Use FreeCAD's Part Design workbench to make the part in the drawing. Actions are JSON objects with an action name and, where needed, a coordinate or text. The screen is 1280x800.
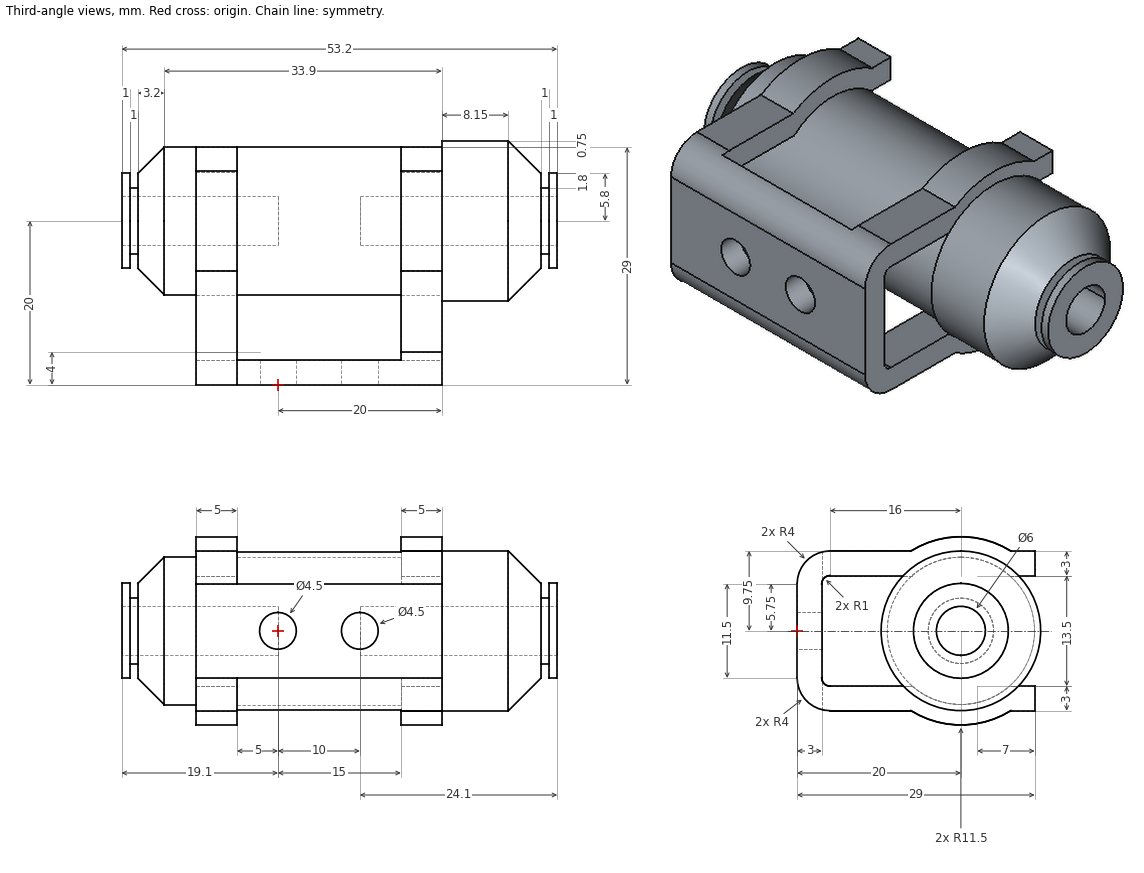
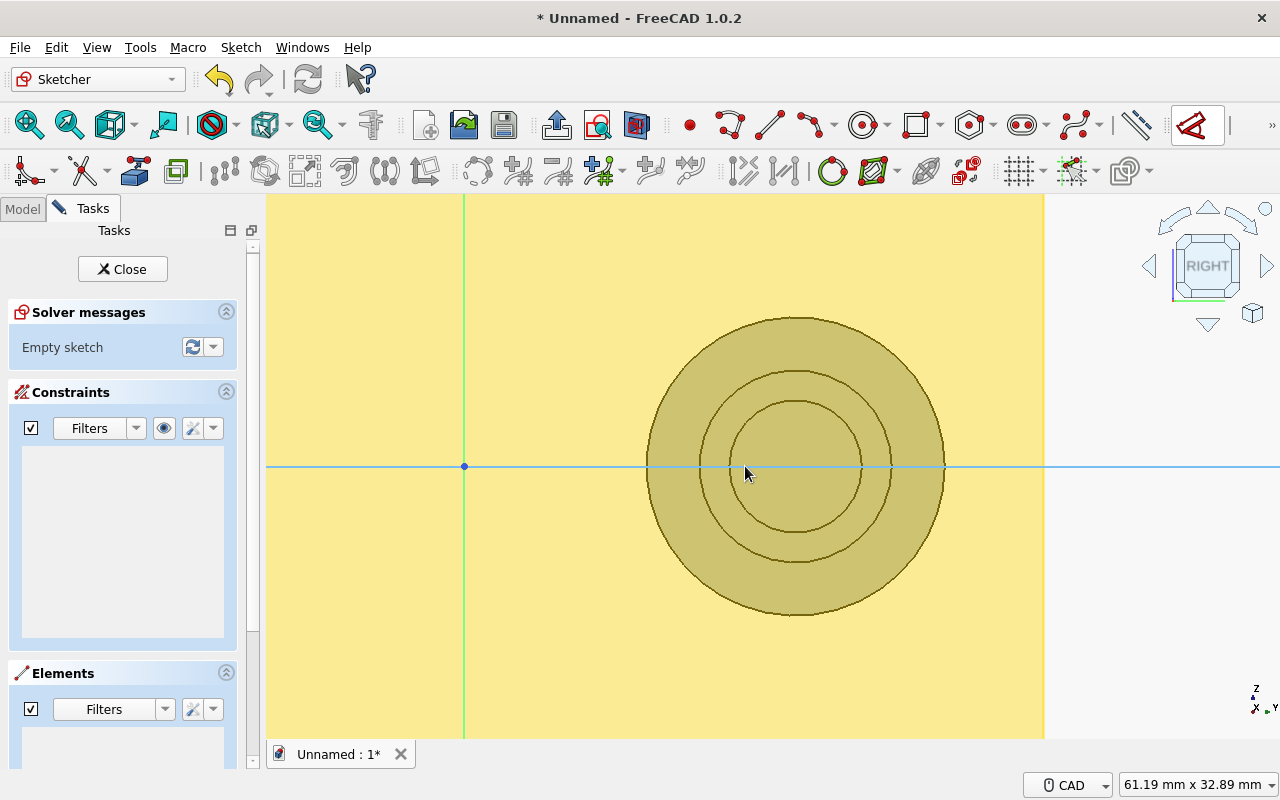
{"action": "left_click", "coordinate": [770, 126]}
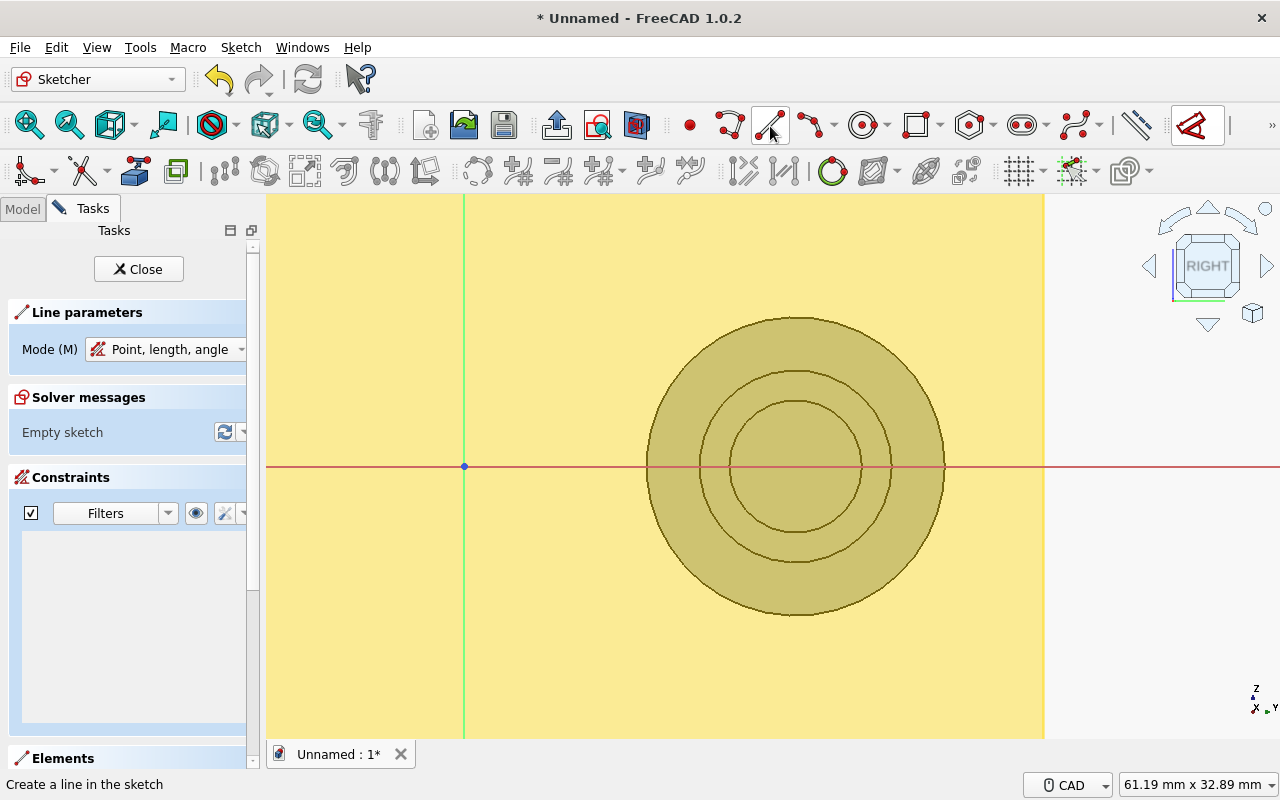
{"action": "left_click", "coordinate": [695, 305]}
{"action": "left_click", "coordinate": [530, 305]}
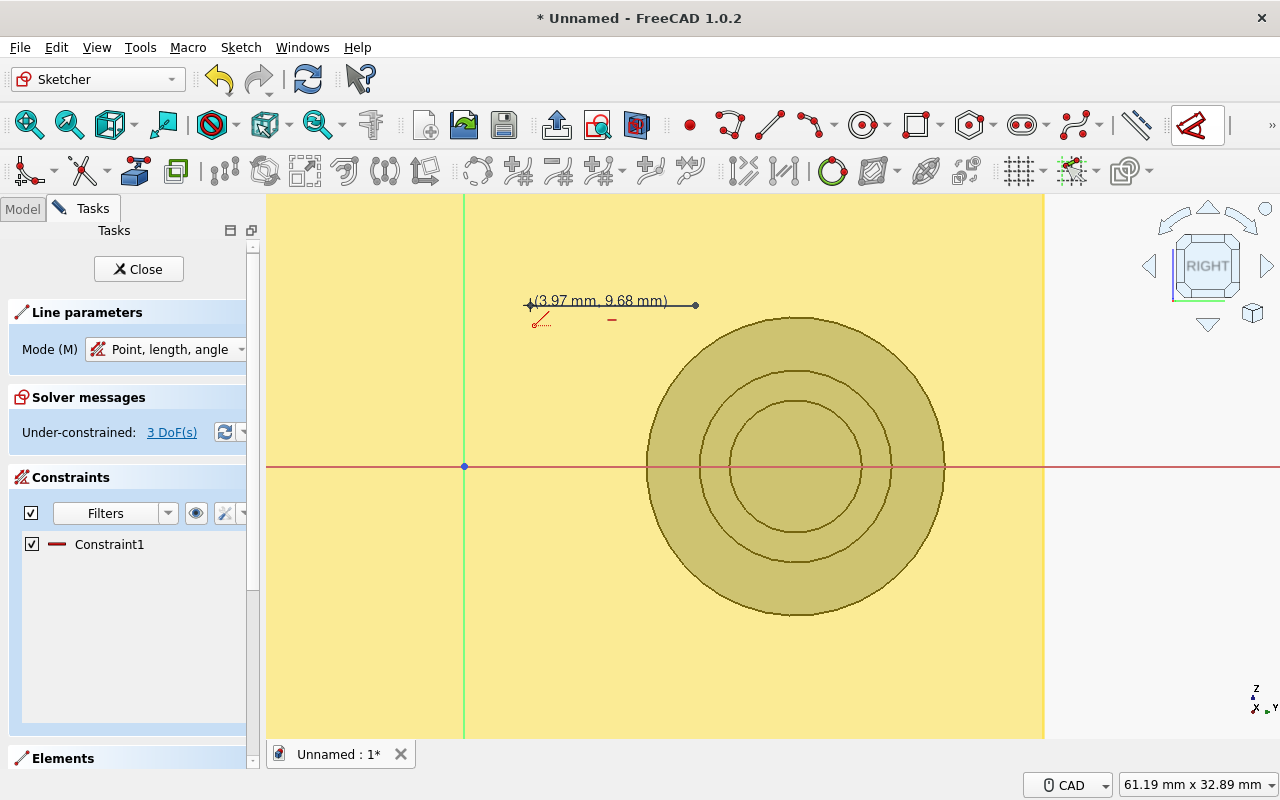
{"action": "left_click", "coordinate": [464, 371]}
{"action": "left_click", "coordinate": [473, 562]}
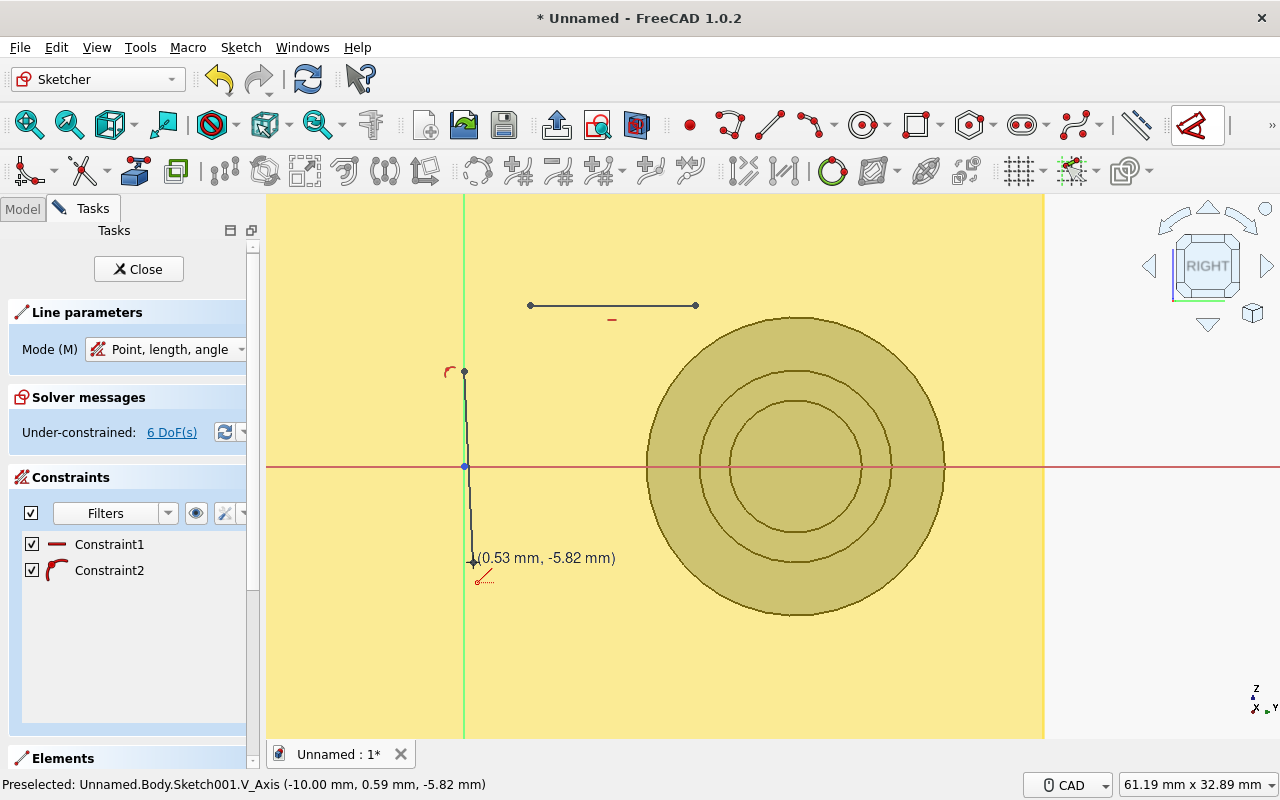
{"action": "left_click", "coordinate": [530, 628]}
{"action": "left_click", "coordinate": [695, 628]}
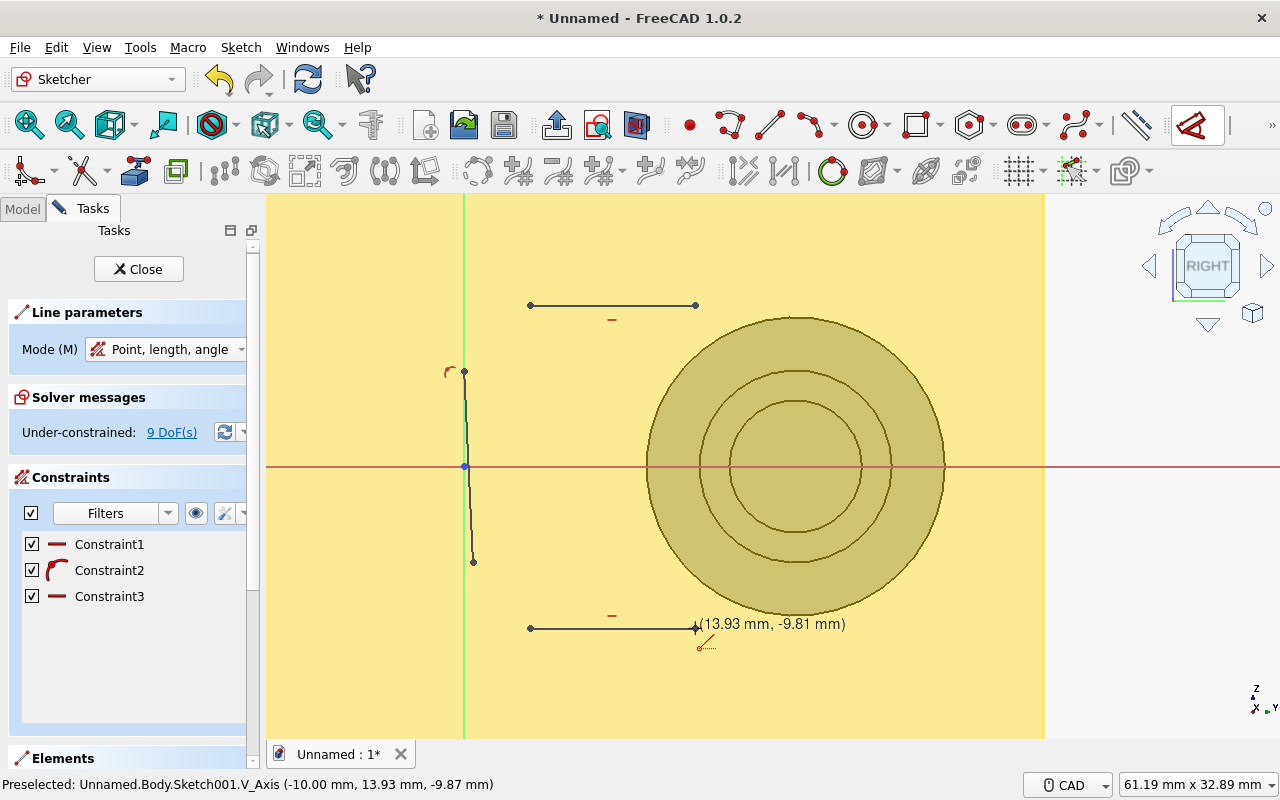
{"action": "left_click", "coordinate": [730, 126]}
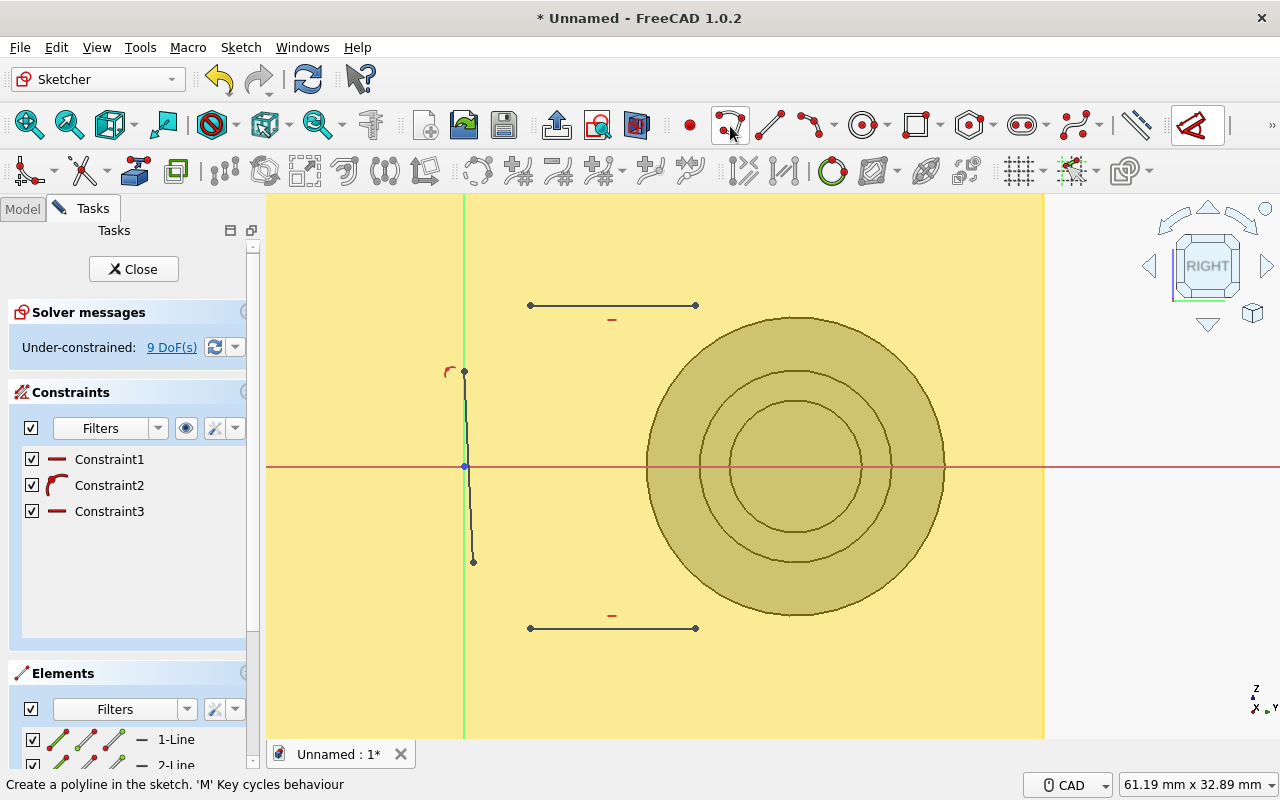
{"action": "left_click", "coordinate": [897, 628]}
{"action": "left_click", "coordinate": [945, 628]}
{"action": "left_click", "coordinate": [945, 578]}
{"action": "left_click", "coordinate": [829, 578]}
{"action": "left_click", "coordinate": [829, 355]}
{"action": "left_click", "coordinate": [945, 355]}
{"action": "left_click", "coordinate": [945, 305]}
{"action": "left_click", "coordinate": [897, 305]}
{"action": "right_click", "coordinate": [897, 305]}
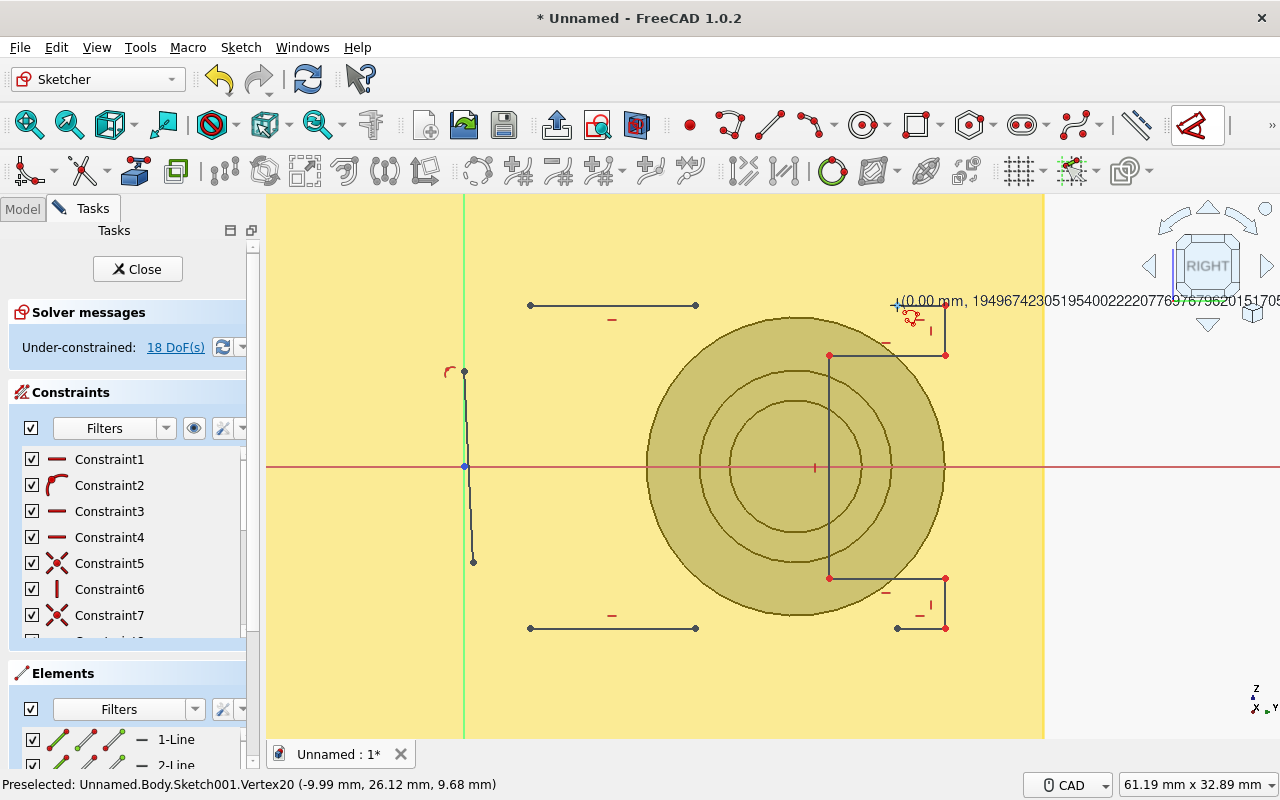
{"action": "left_click", "coordinate": [810, 126]}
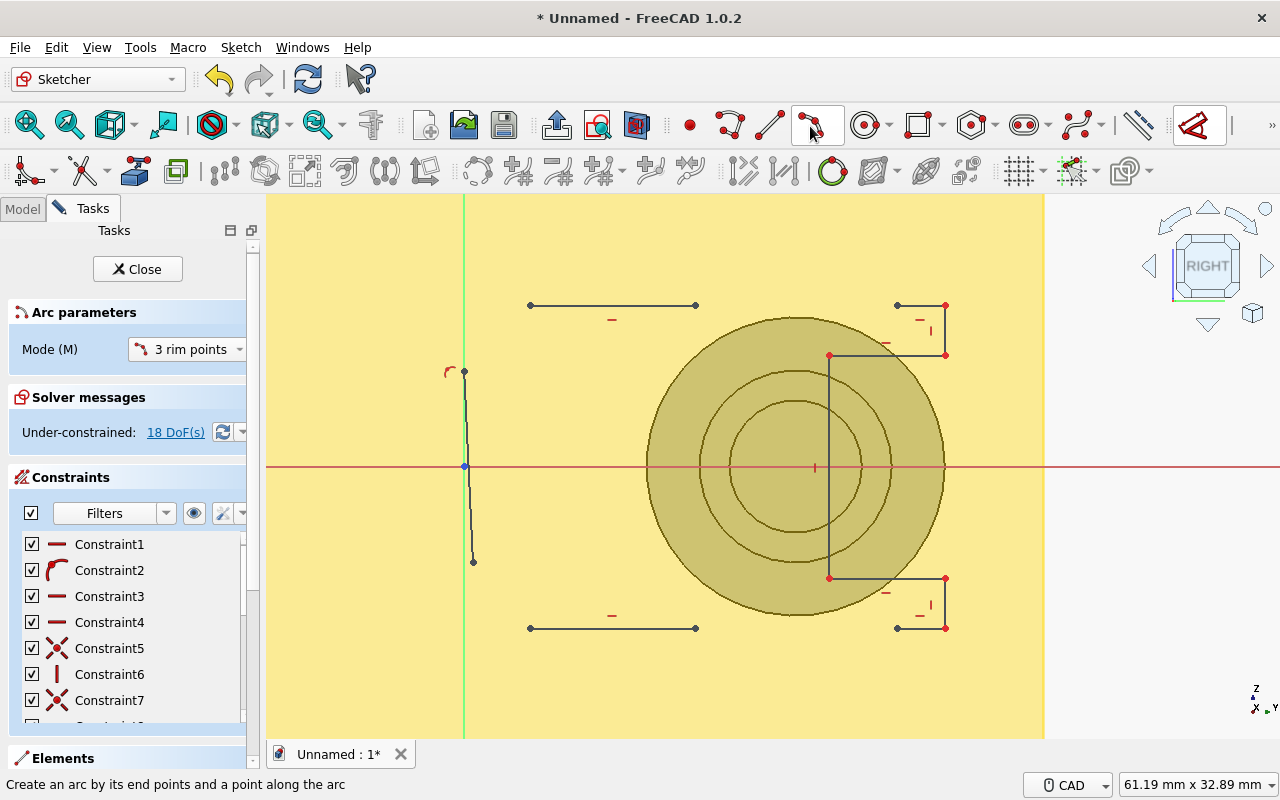
{"action": "left_click", "coordinate": [530, 306]}
{"action": "left_click", "coordinate": [464, 372]}
{"action": "left_click", "coordinate": [484, 324]}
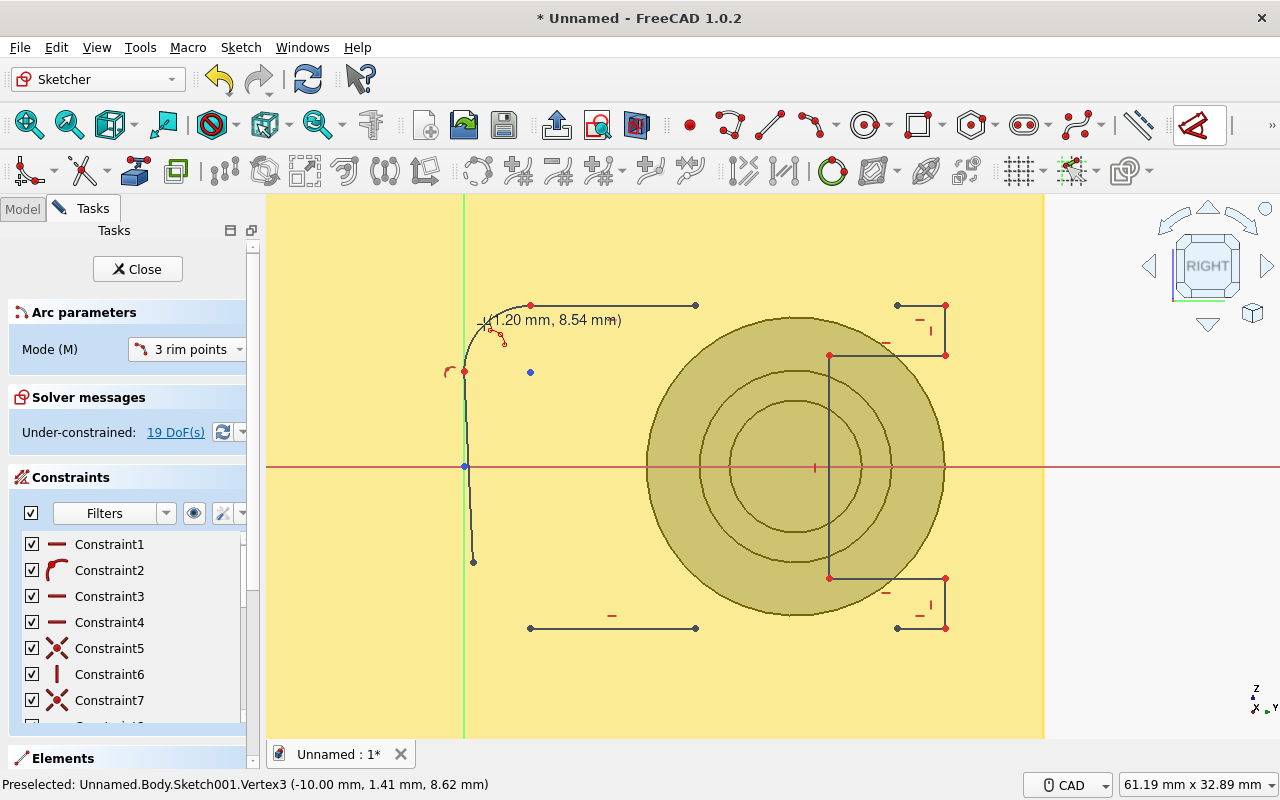
{"action": "left_click", "coordinate": [473, 563]}
{"action": "left_click", "coordinate": [530, 629]}
{"action": "left_click", "coordinate": [484, 609]}